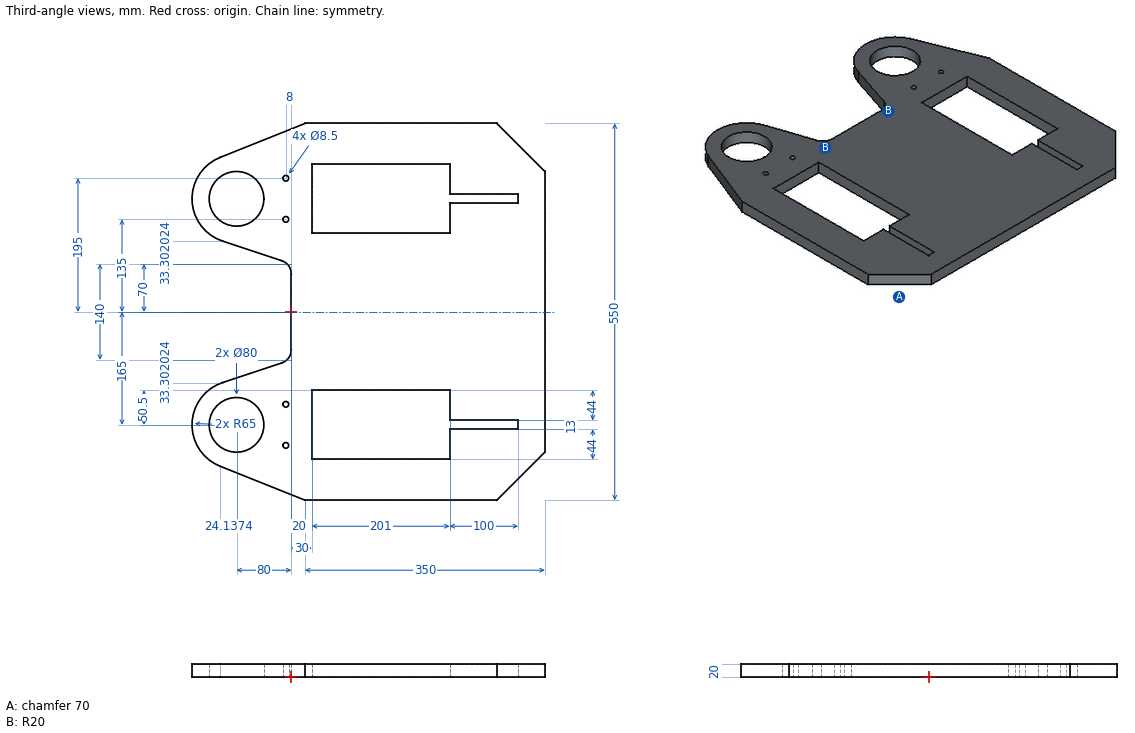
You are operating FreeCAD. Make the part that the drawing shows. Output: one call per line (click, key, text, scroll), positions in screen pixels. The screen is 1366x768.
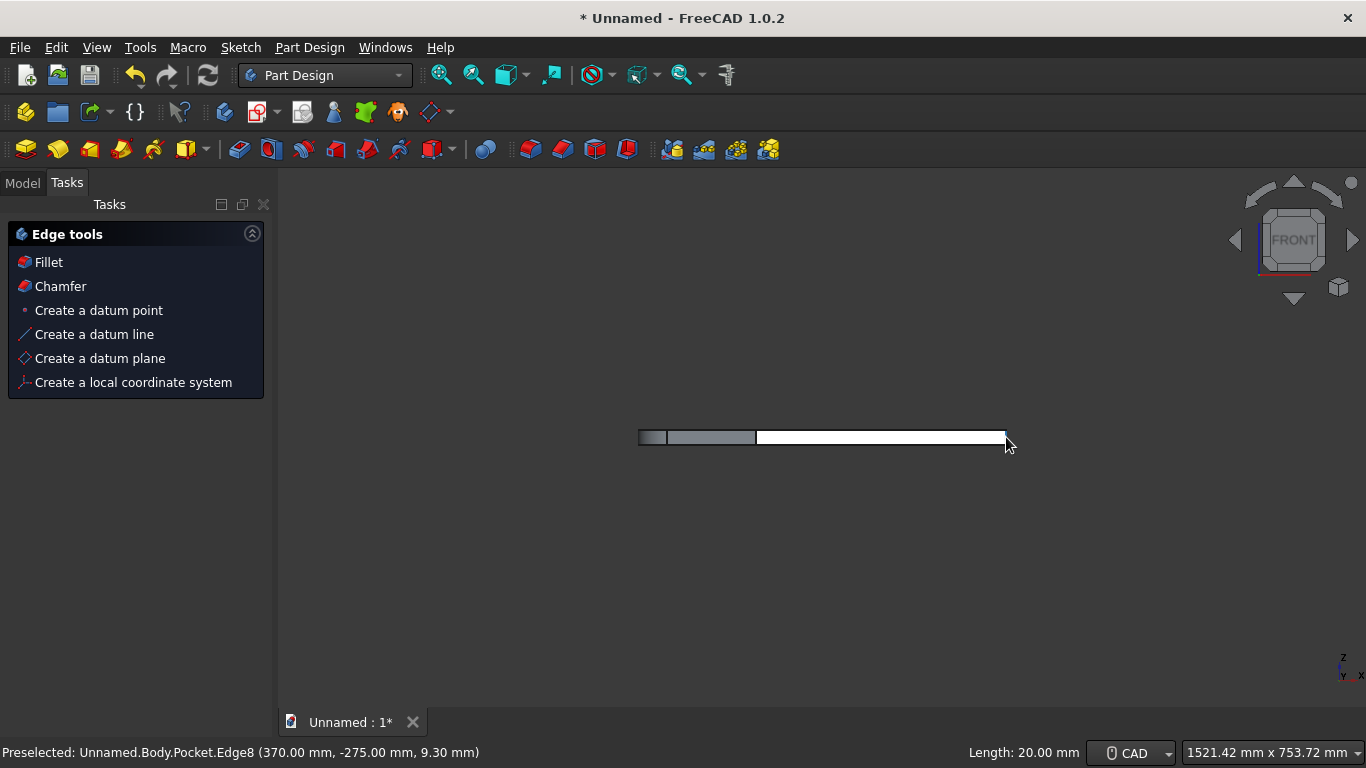
key(3)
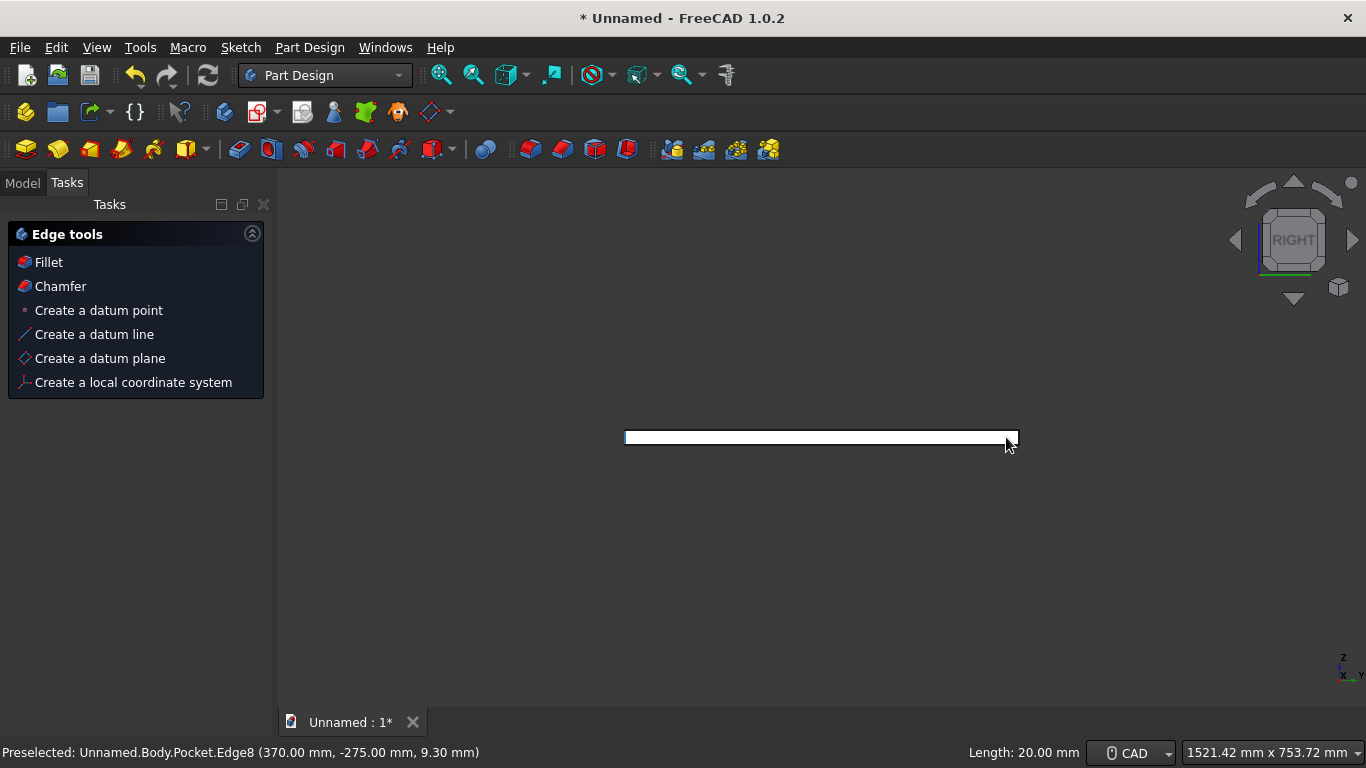
click(442, 76)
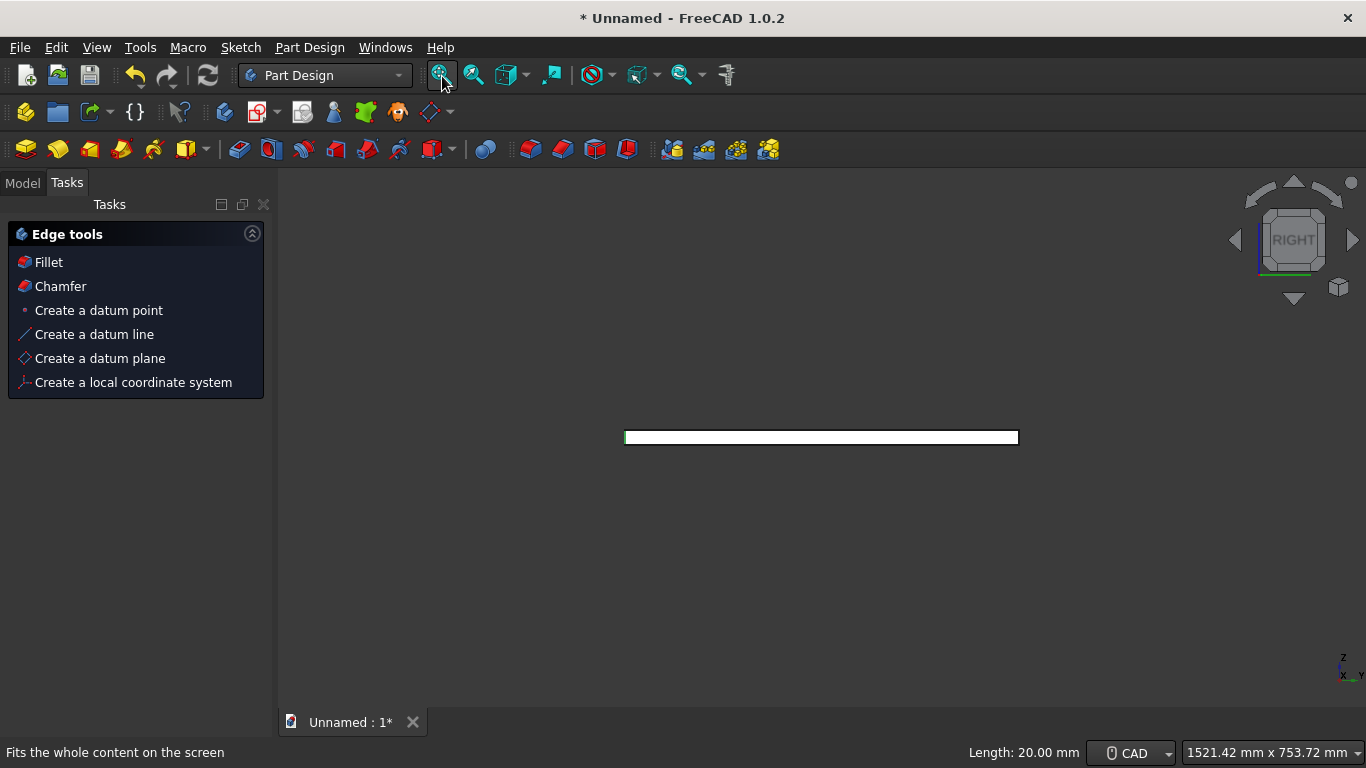
click(1019, 436, ctrl)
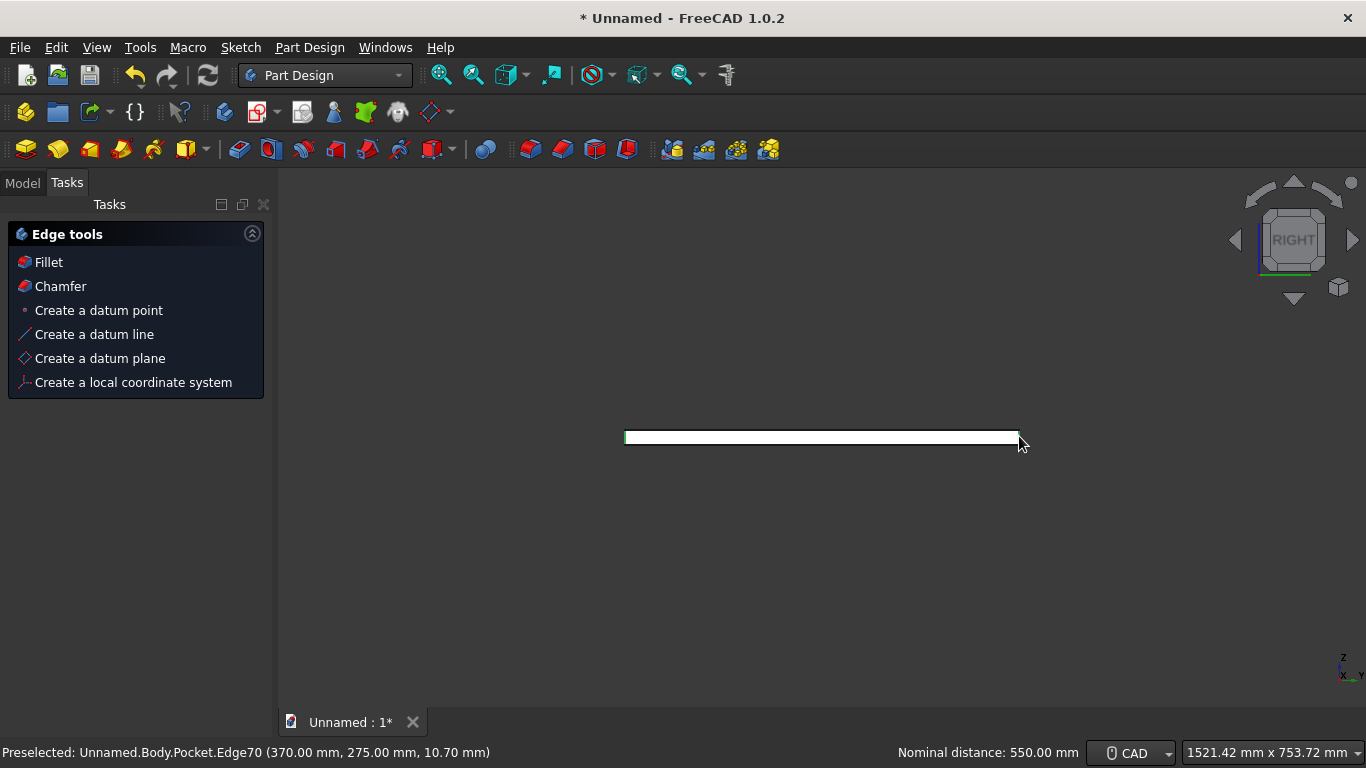
click(564, 150)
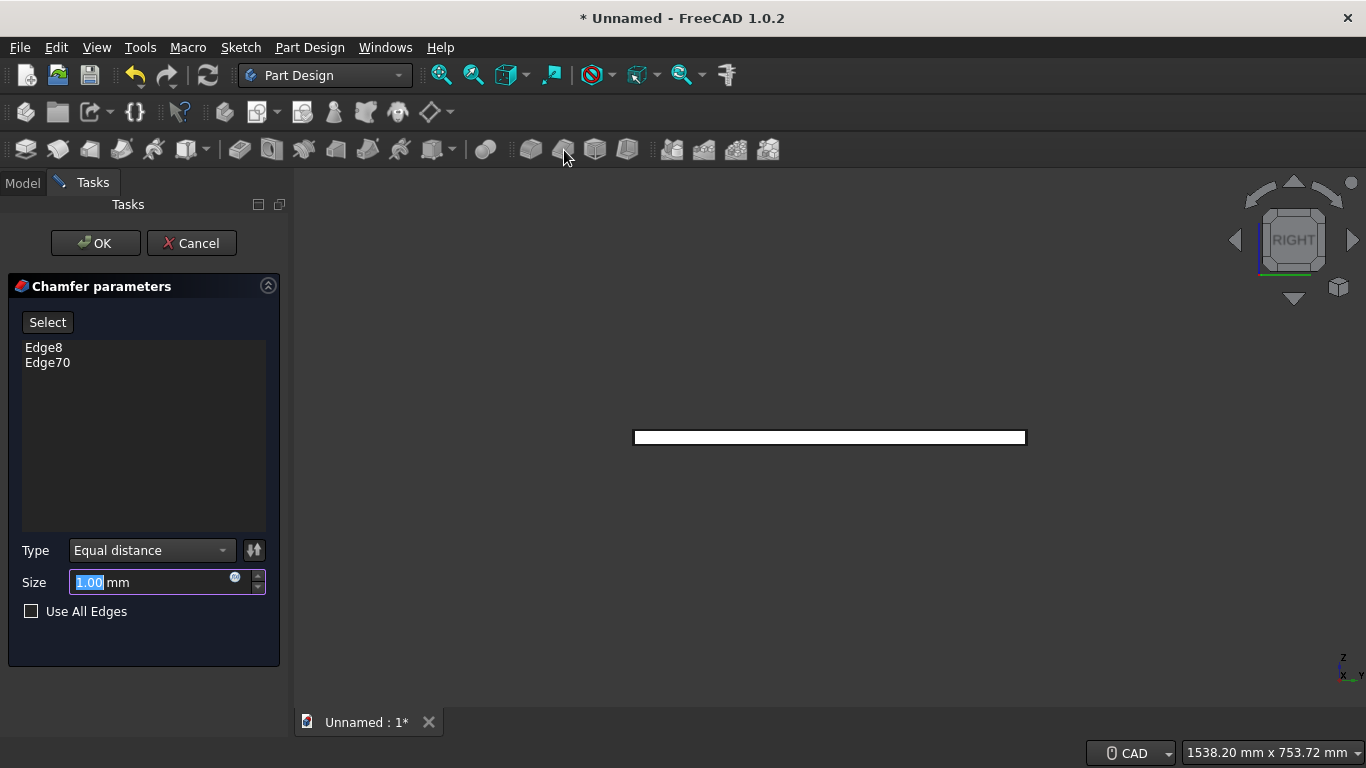
text(70)
key(Tab)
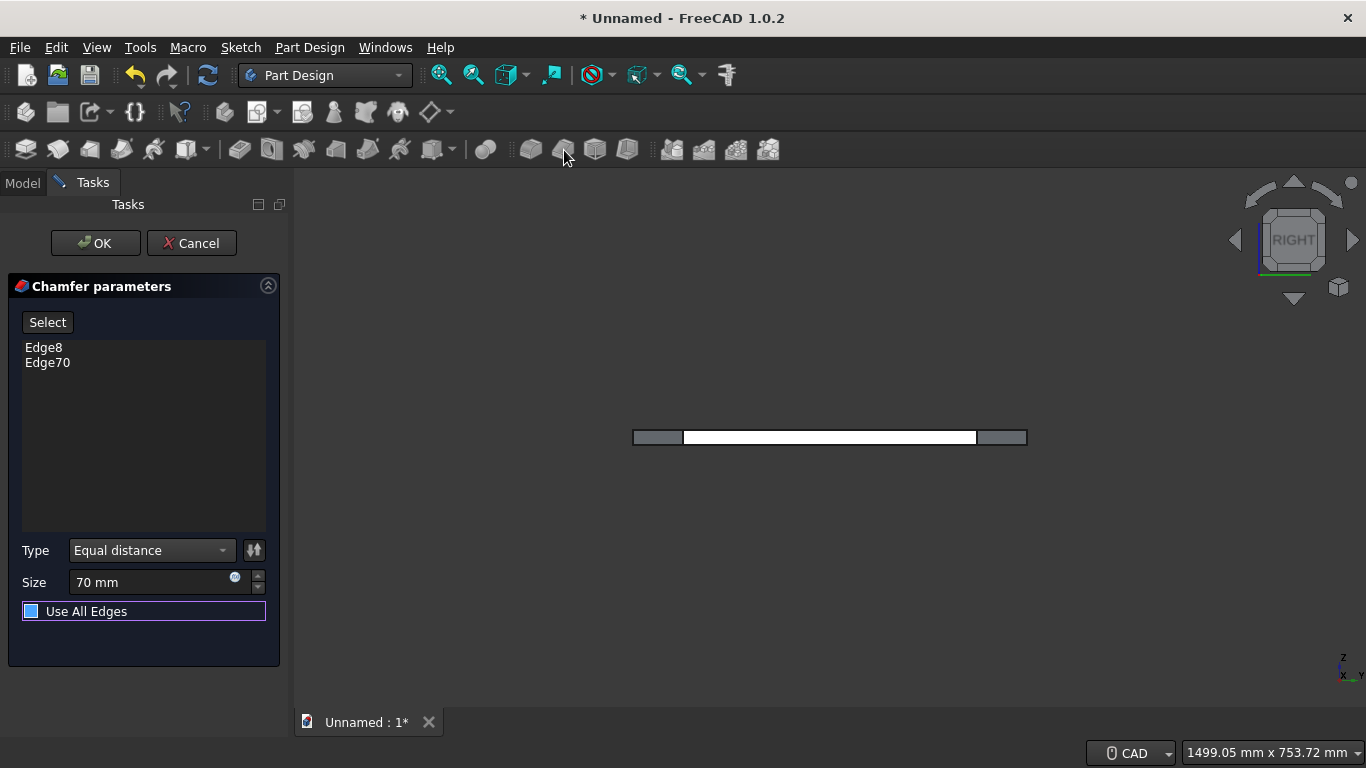
click(96, 243)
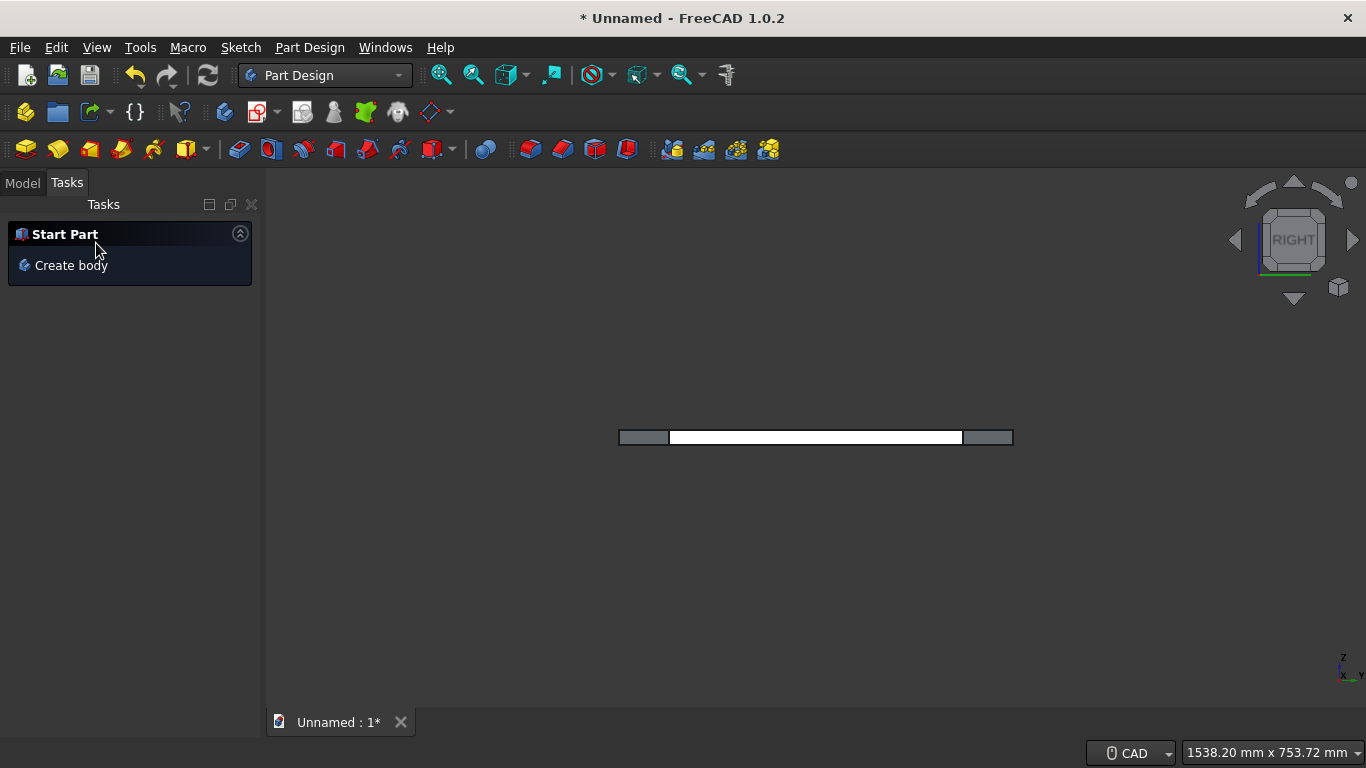
key(v)
key(f)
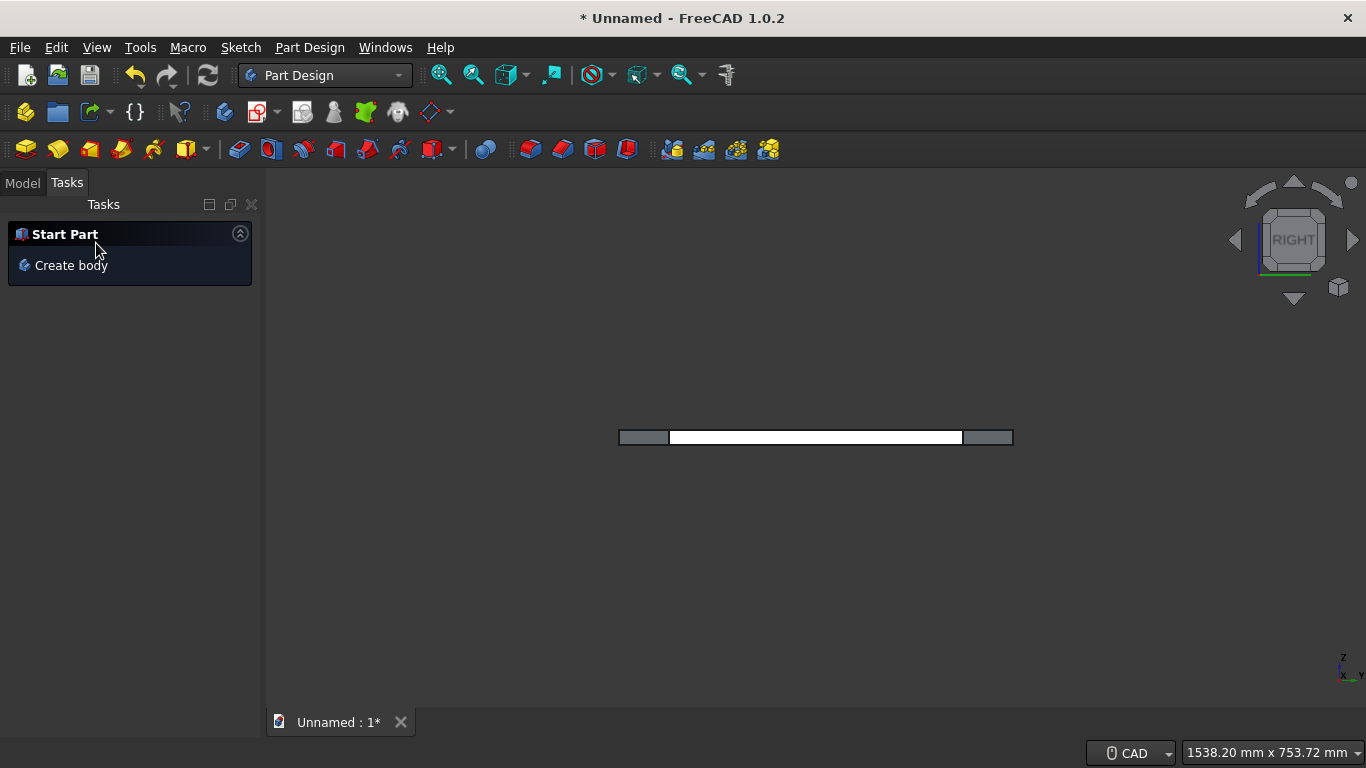
scroll(766, 436, up, 6)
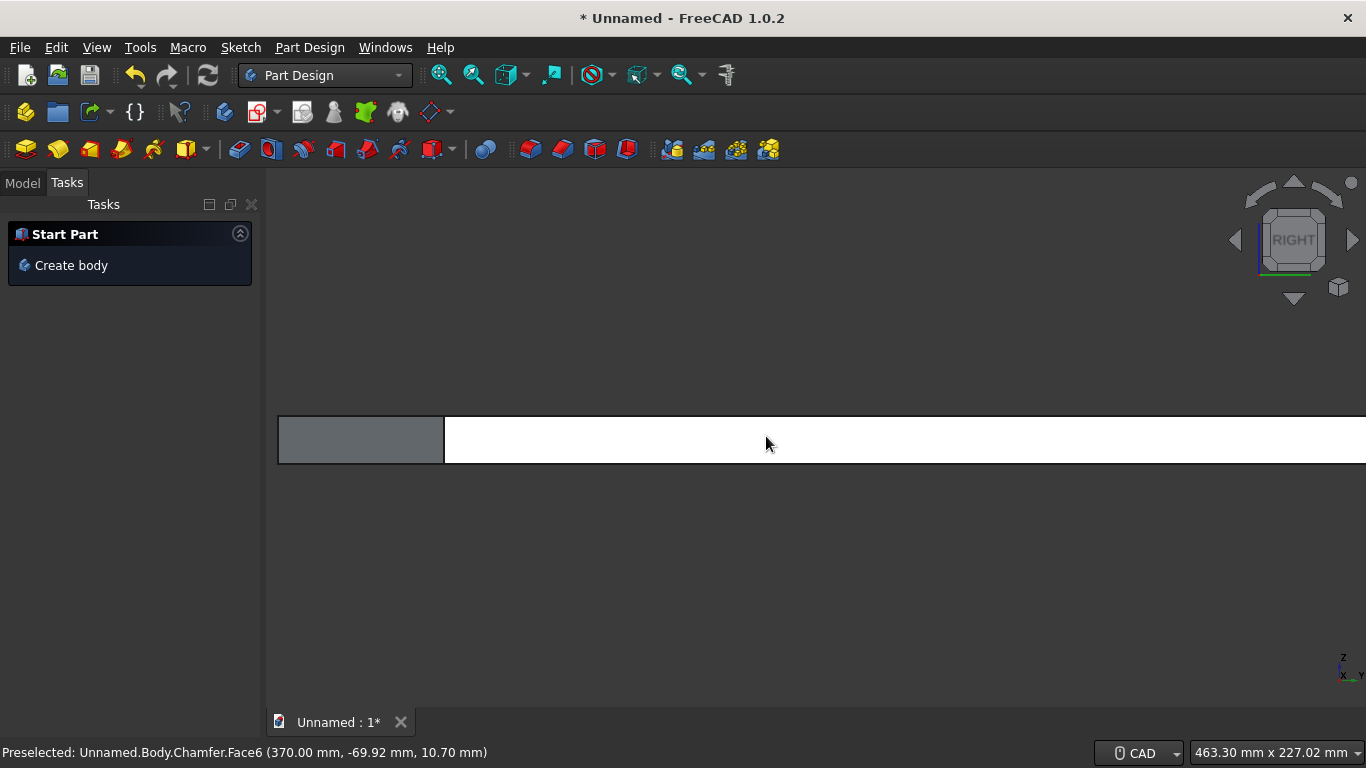
key(v)
key(f)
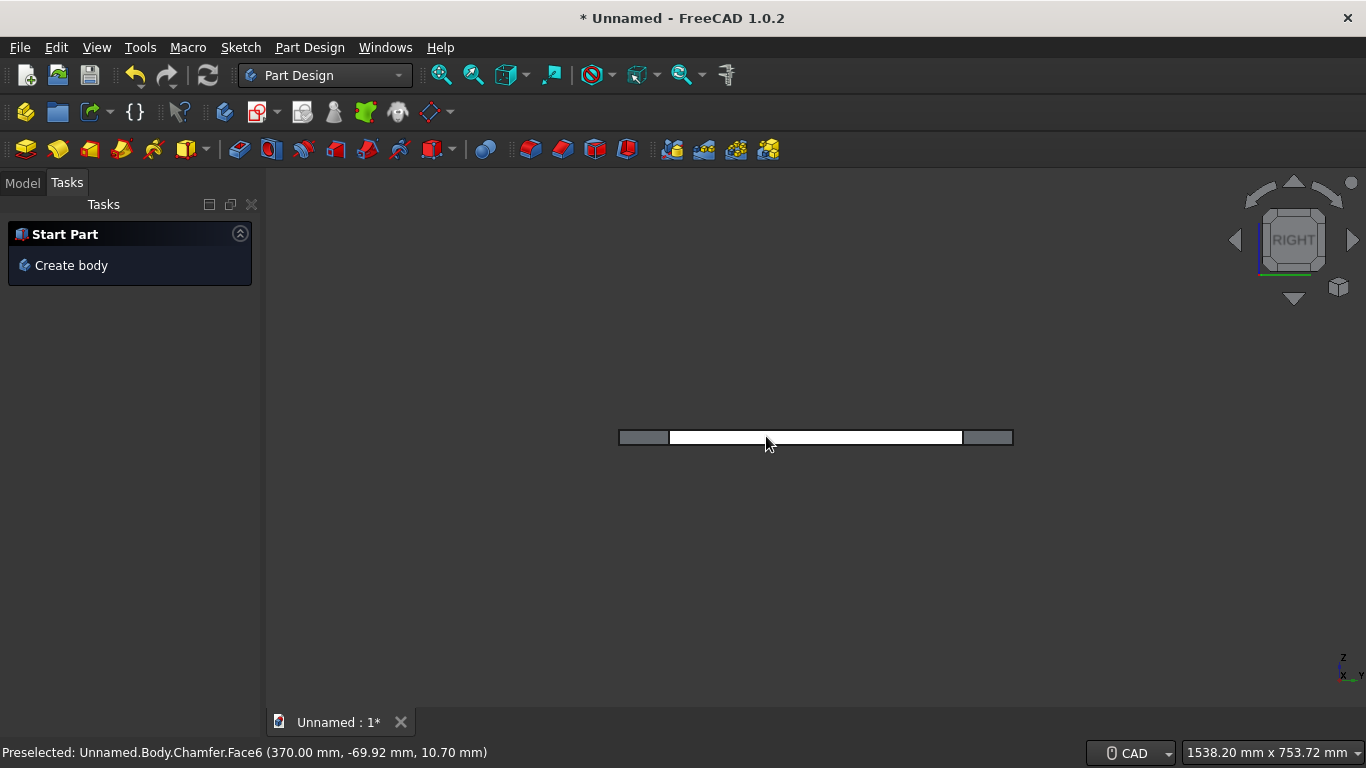
key(0)